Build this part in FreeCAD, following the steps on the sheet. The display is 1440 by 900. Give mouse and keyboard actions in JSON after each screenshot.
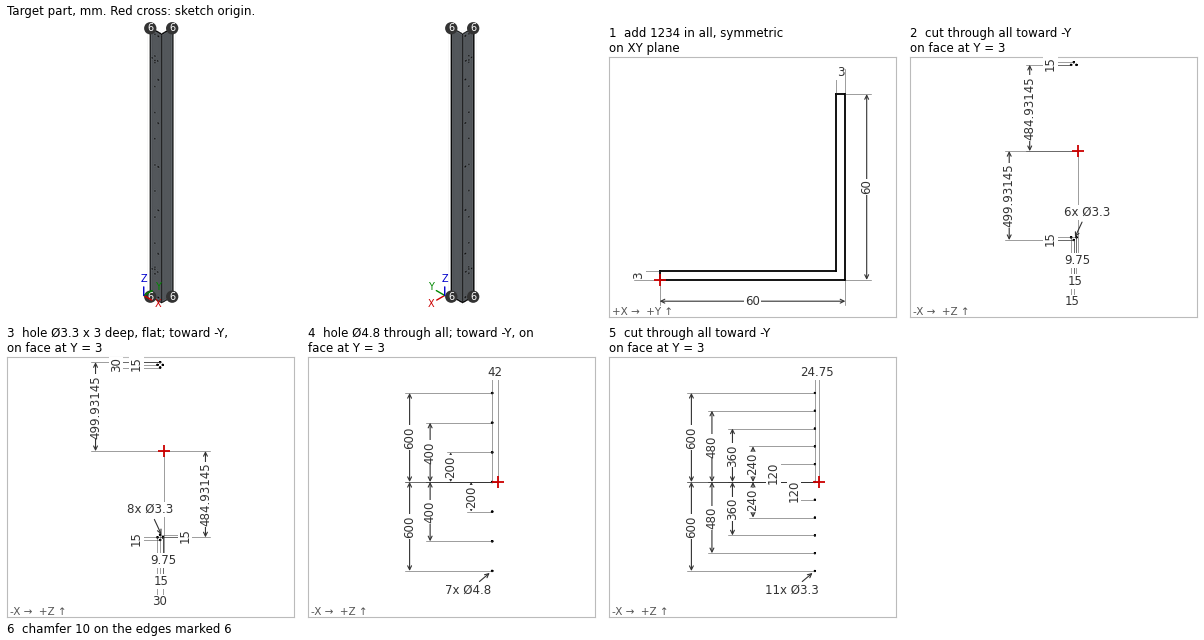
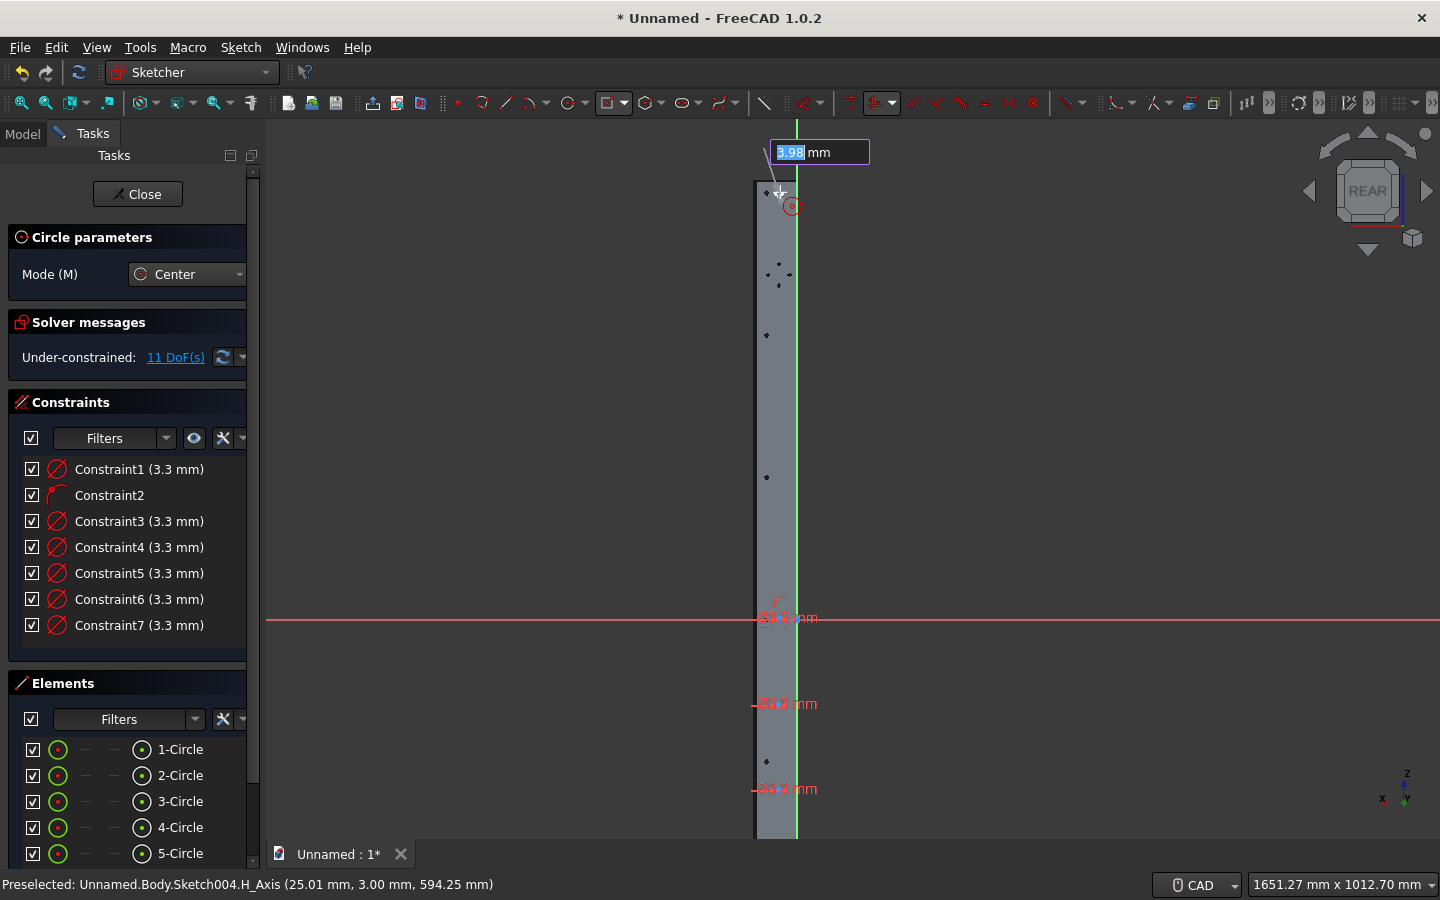
{"action": "type", "text": "3.3"}
{"action": "key", "text": "Return"}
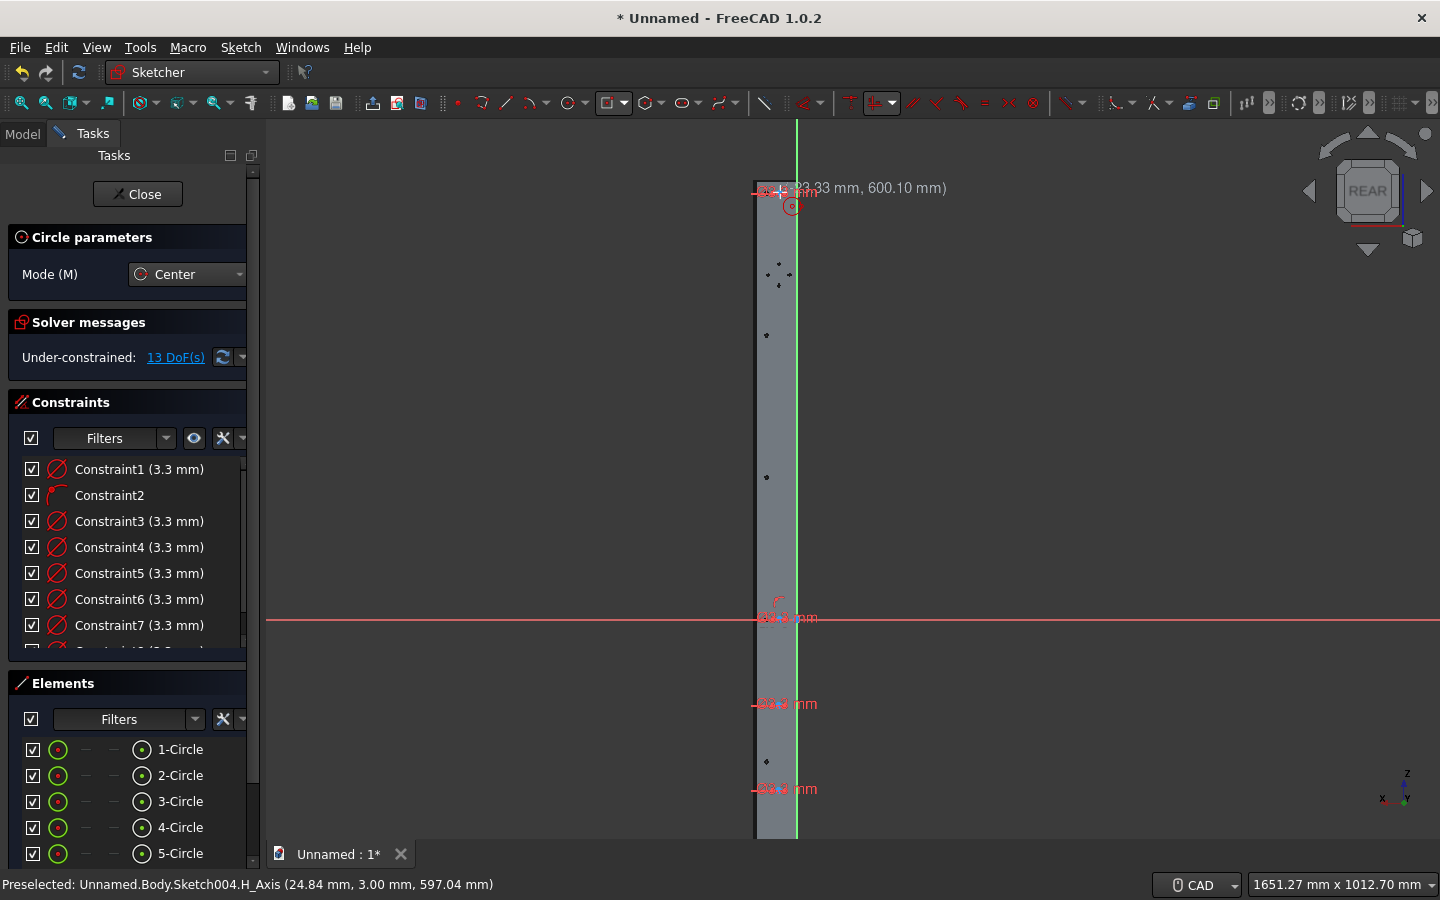
{"action": "scroll", "coordinate": [779, 278], "scroll_direction": "up", "scroll_amount": 15}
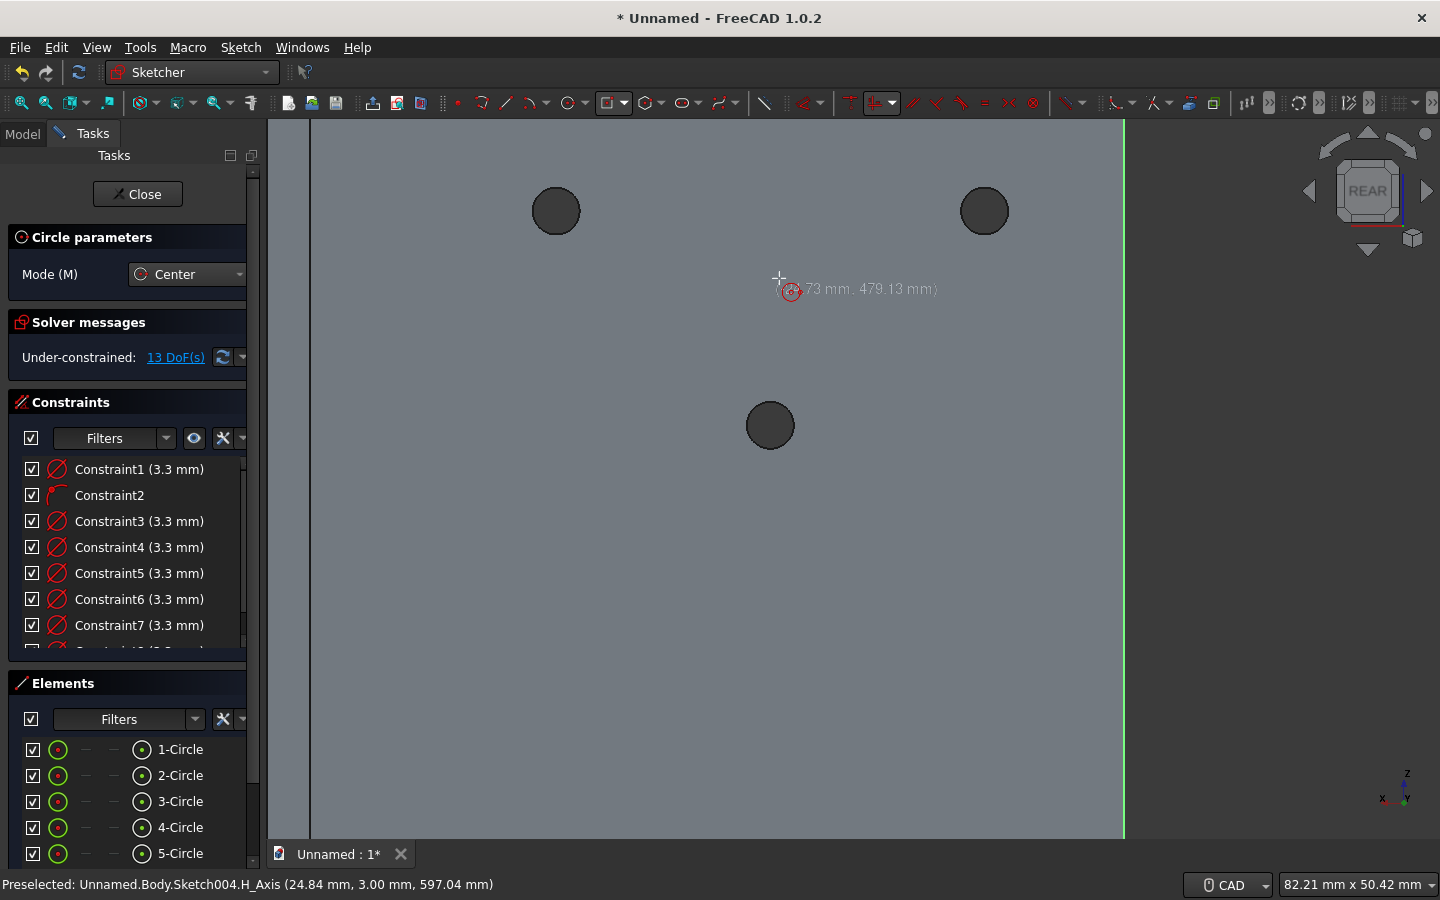
{"action": "scroll", "coordinate": [779, 249], "scroll_direction": "down", "scroll_amount": 17}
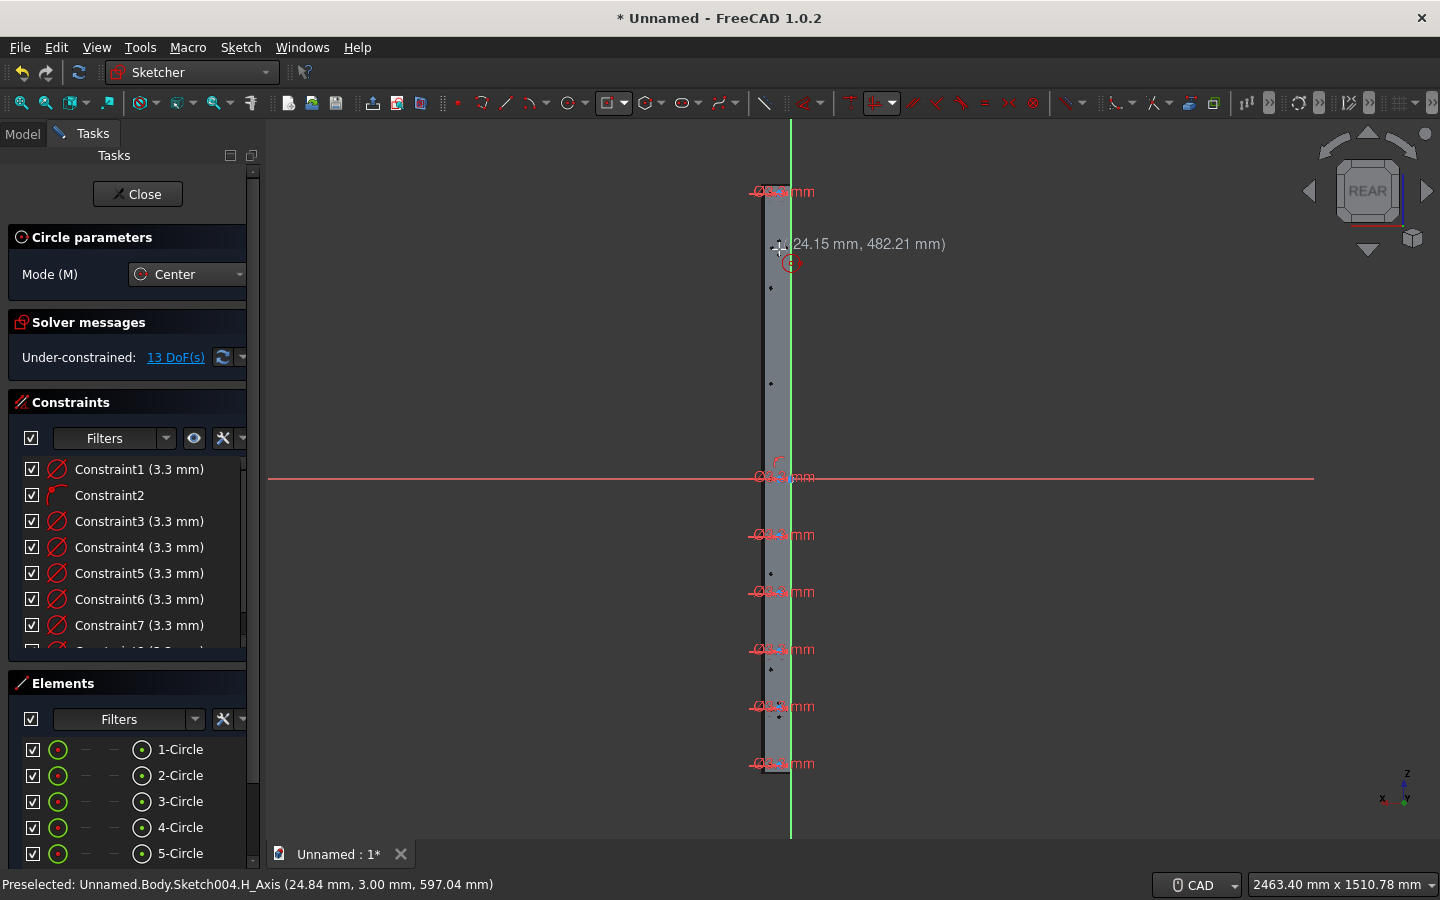
{"action": "scroll", "coordinate": [779, 250], "scroll_direction": "up", "scroll_amount": 2}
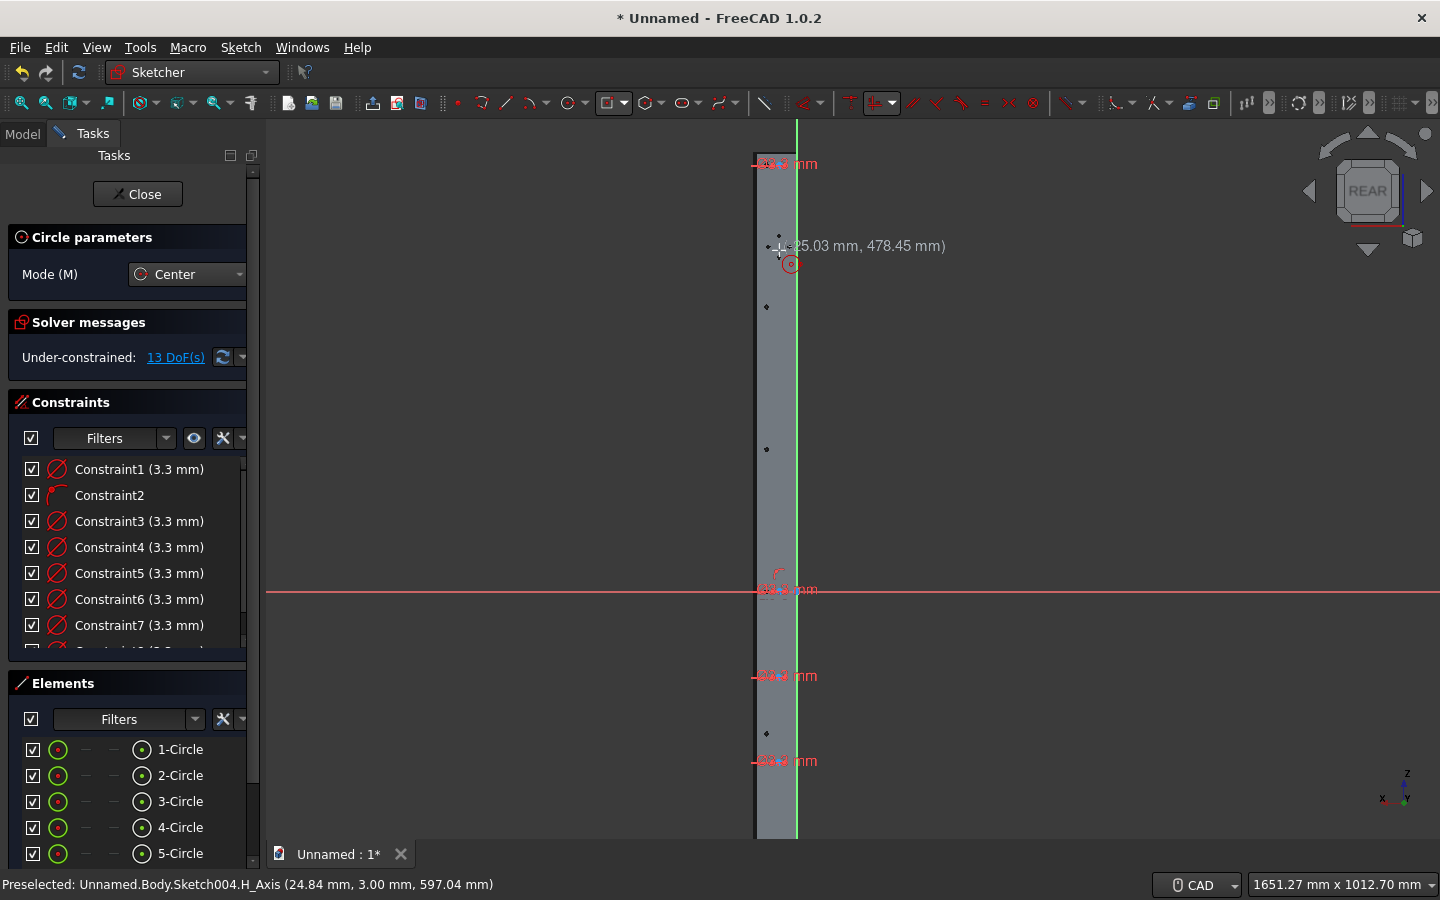
{"action": "left_click", "coordinate": [779, 250]}
{"action": "mouse_move", "coordinate": [780, 249]}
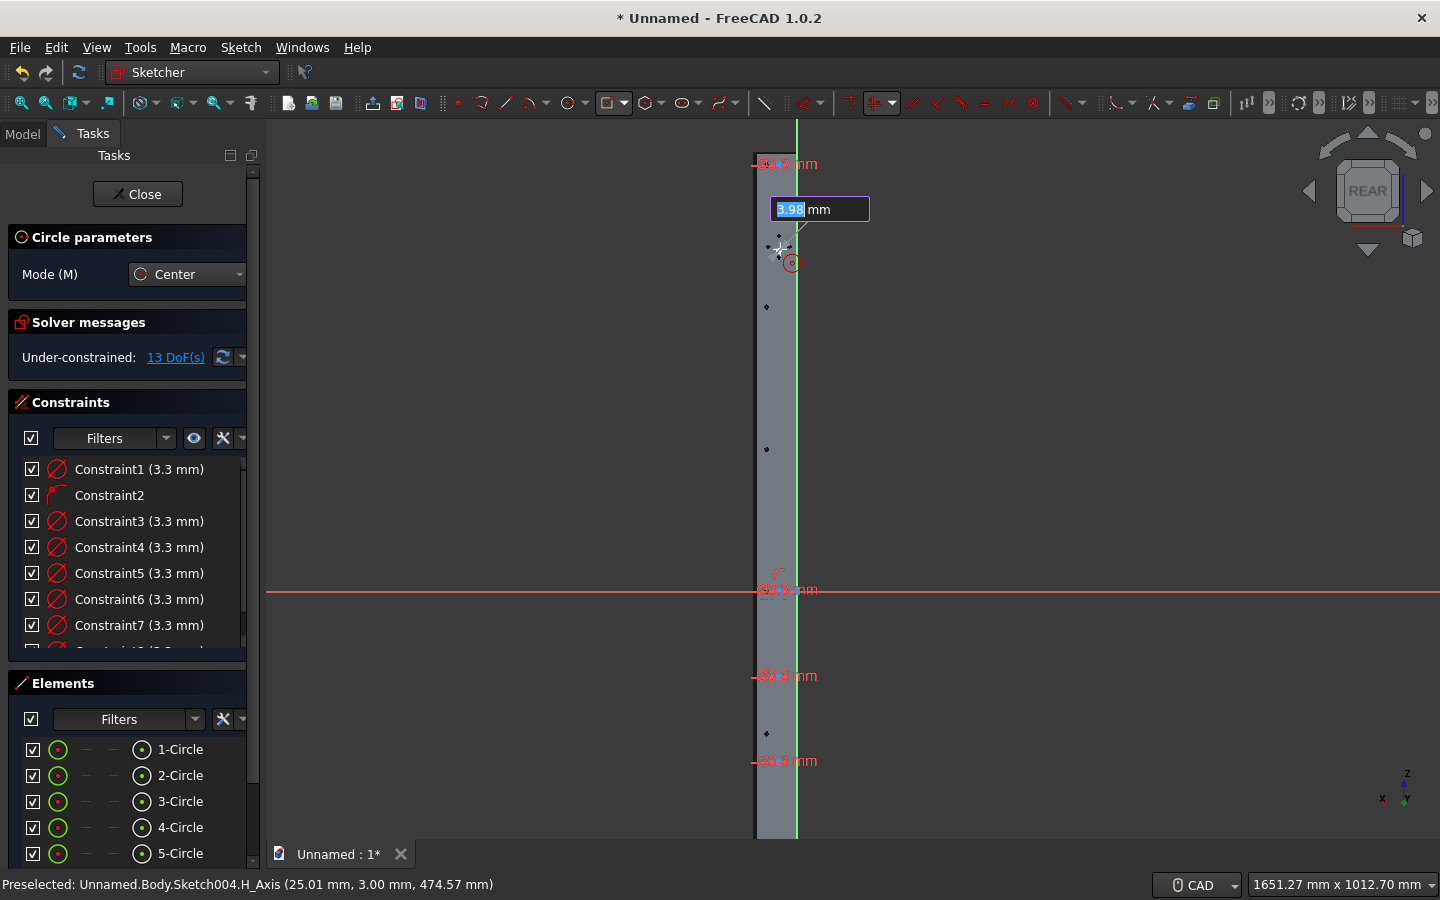
{"action": "type", "text": "3.3"}
{"action": "key", "text": "Return"}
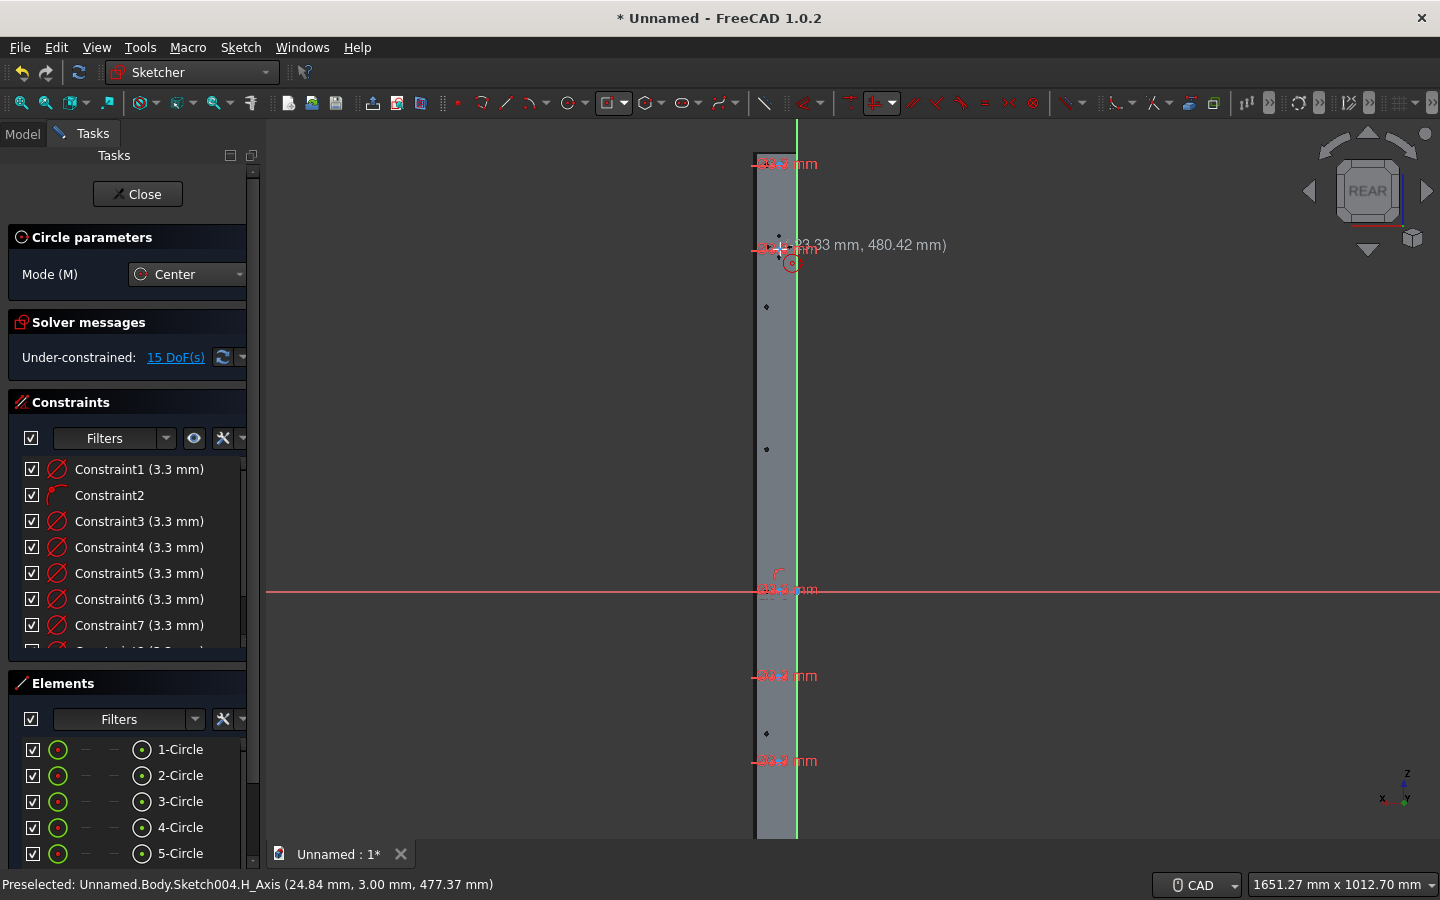
{"action": "scroll", "coordinate": [779, 336], "scroll_direction": "up", "scroll_amount": 15}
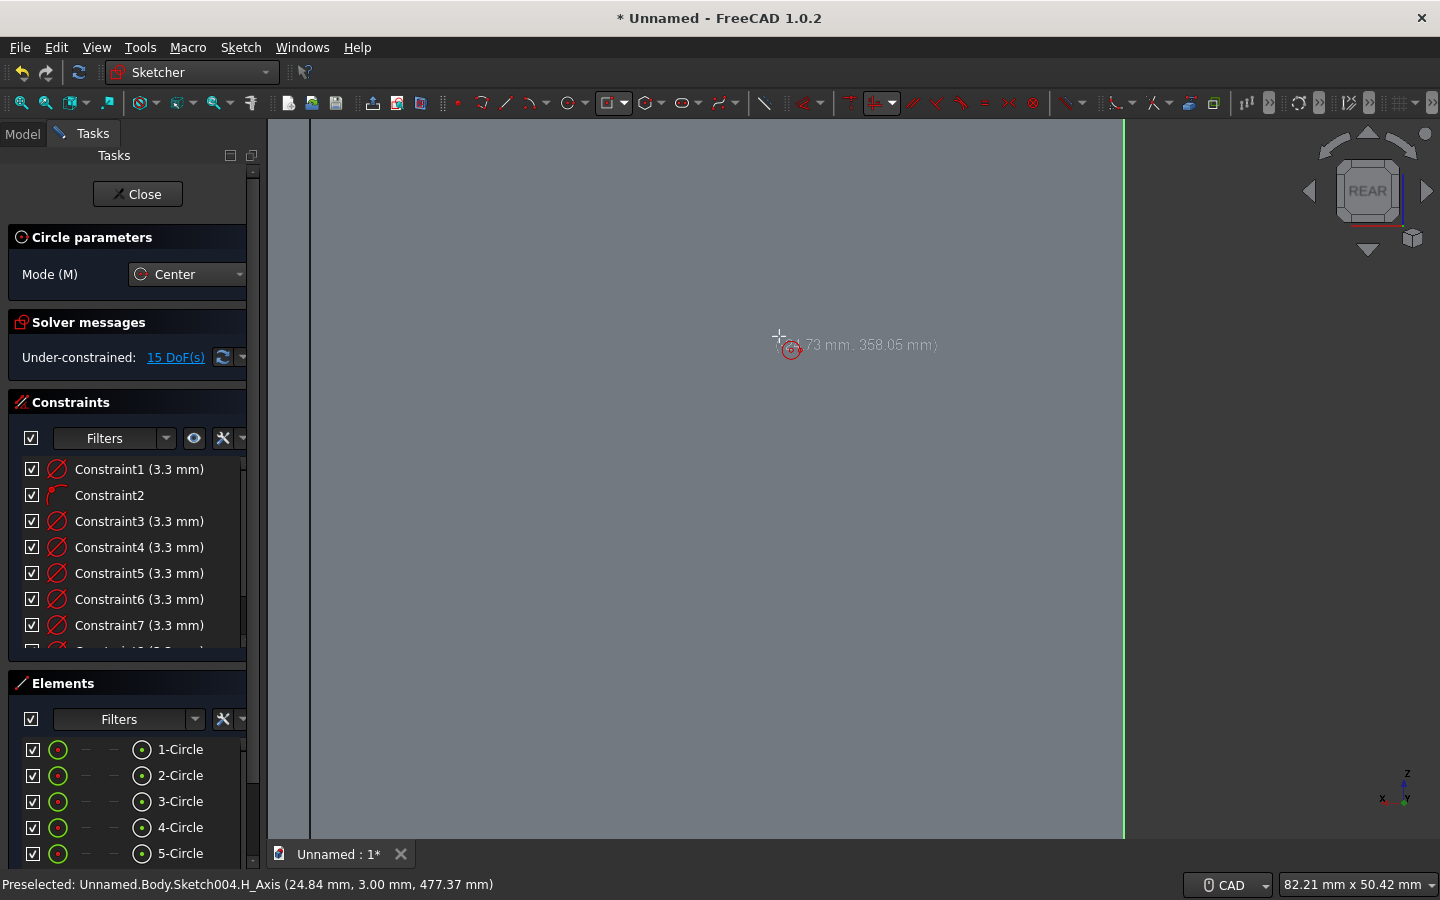
{"action": "scroll", "coordinate": [779, 307], "scroll_direction": "down", "scroll_amount": 17}